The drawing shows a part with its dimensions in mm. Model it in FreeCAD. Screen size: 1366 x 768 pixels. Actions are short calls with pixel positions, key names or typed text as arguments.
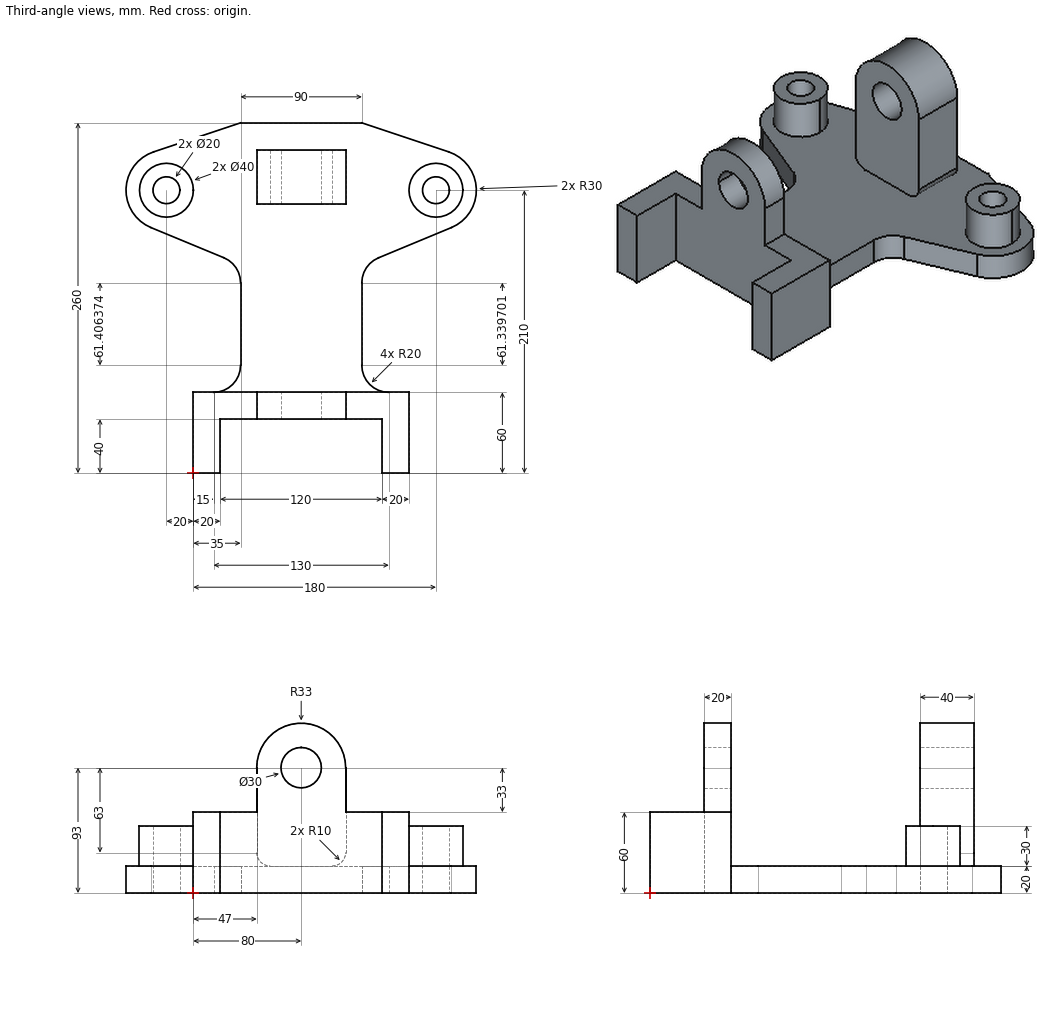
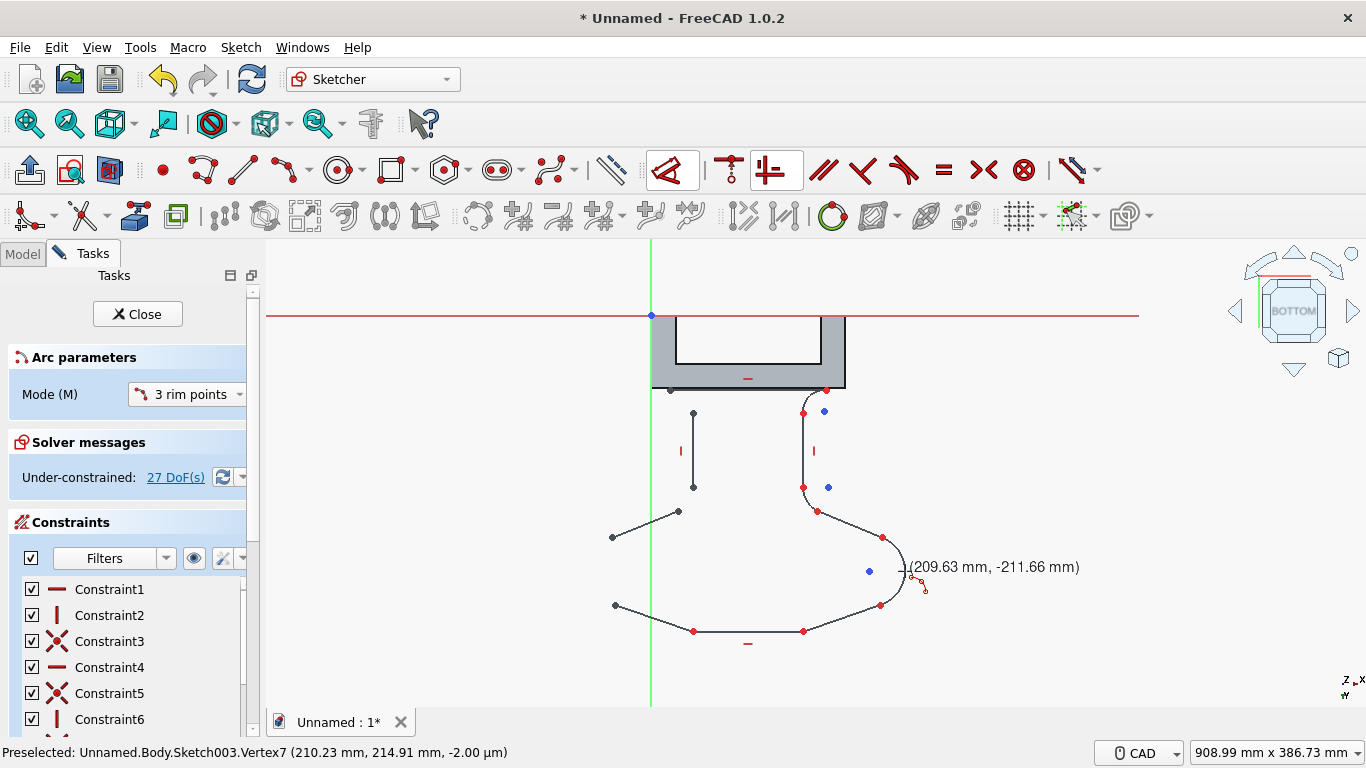
click(615, 605)
click(613, 538)
click(591, 571)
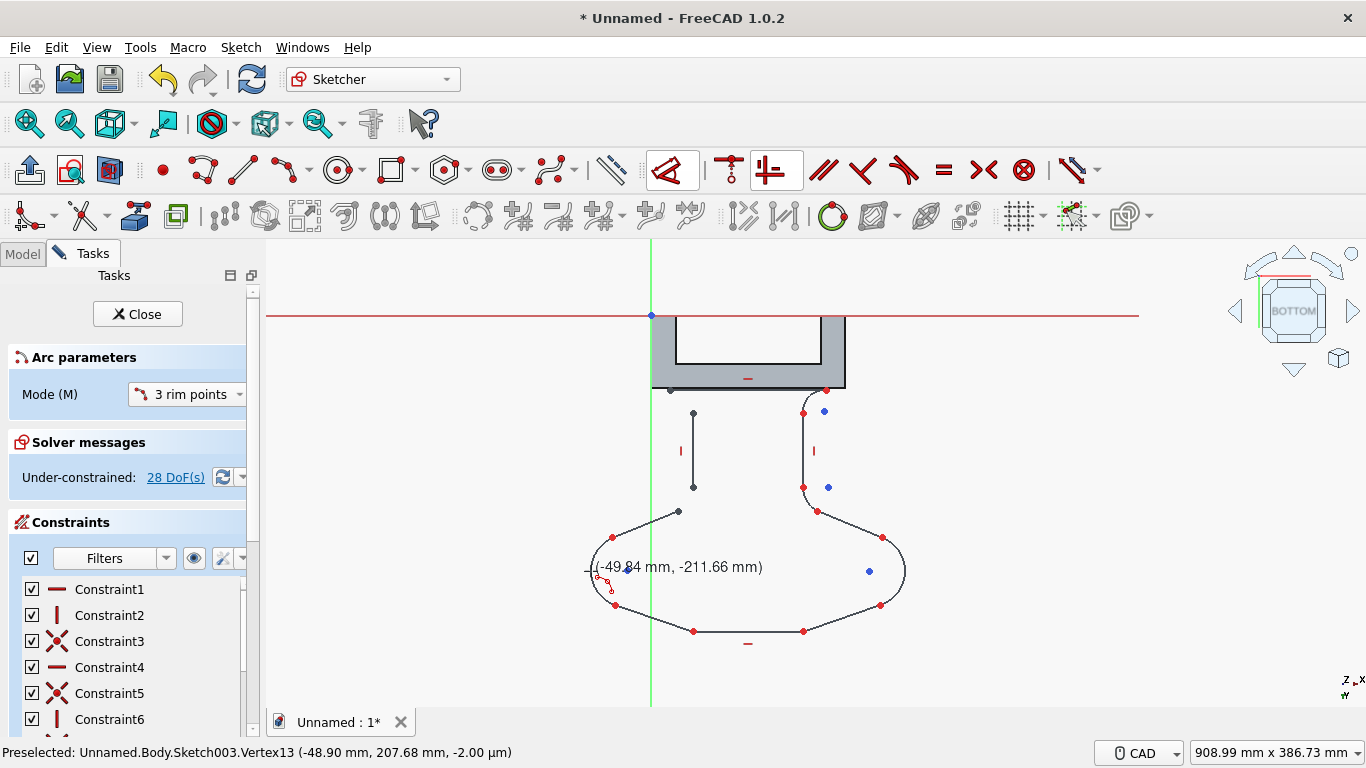
click(679, 511)
click(693, 488)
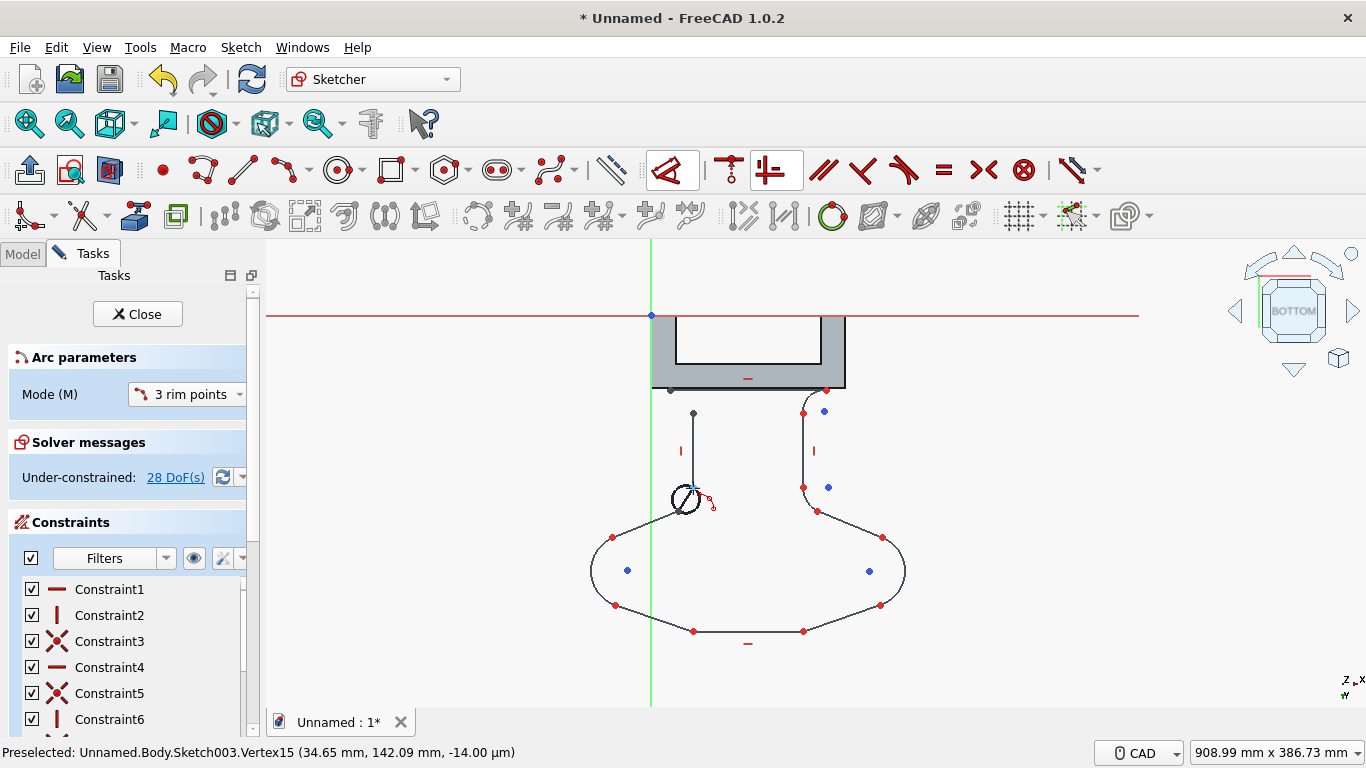
scroll(690, 500, up, 7)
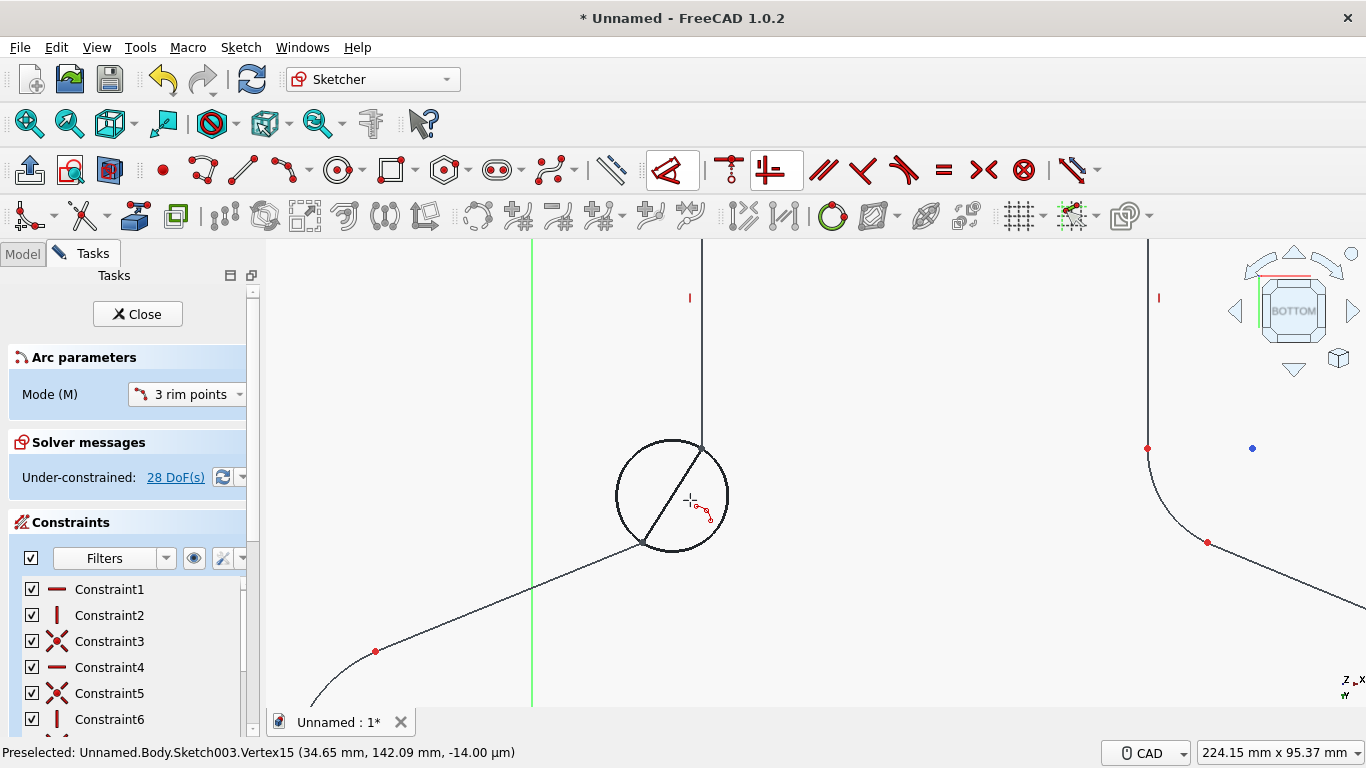
click(687, 500)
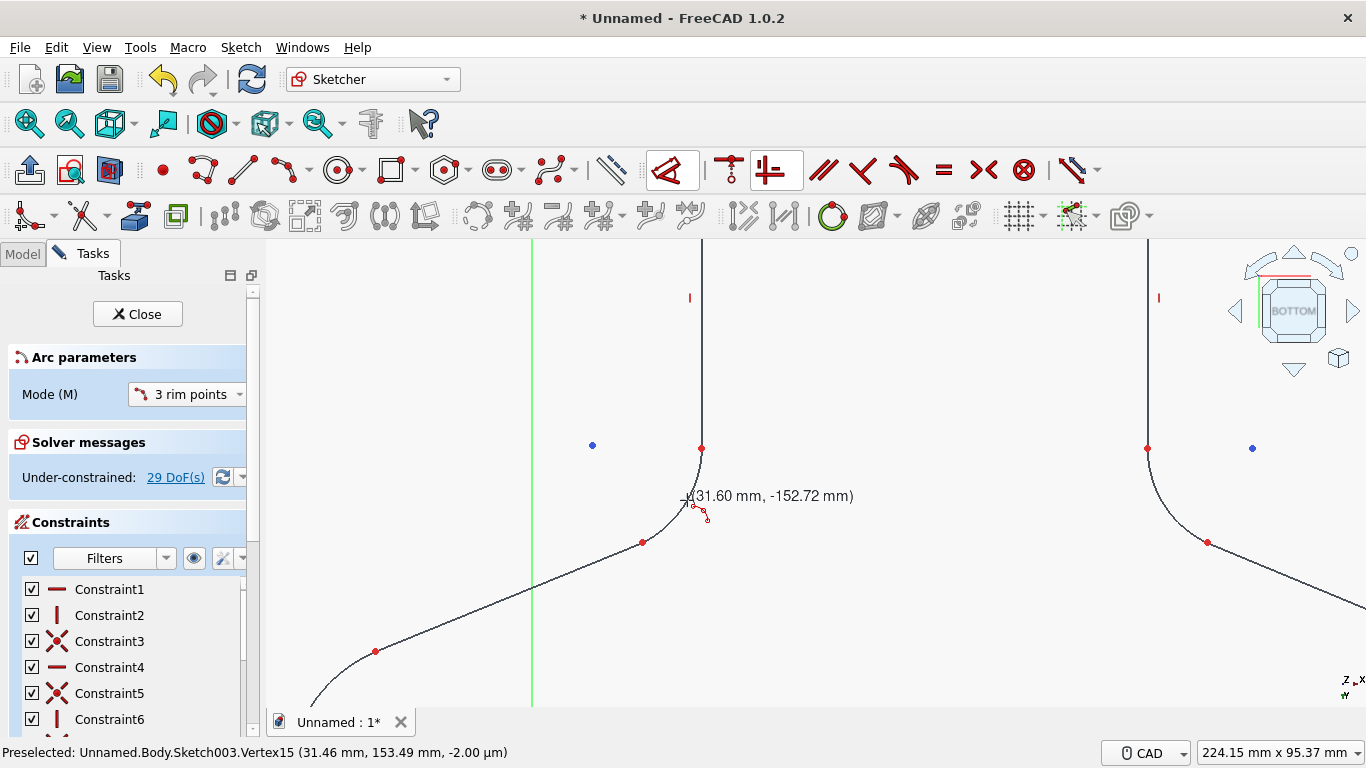
scroll(690, 500, down, 7)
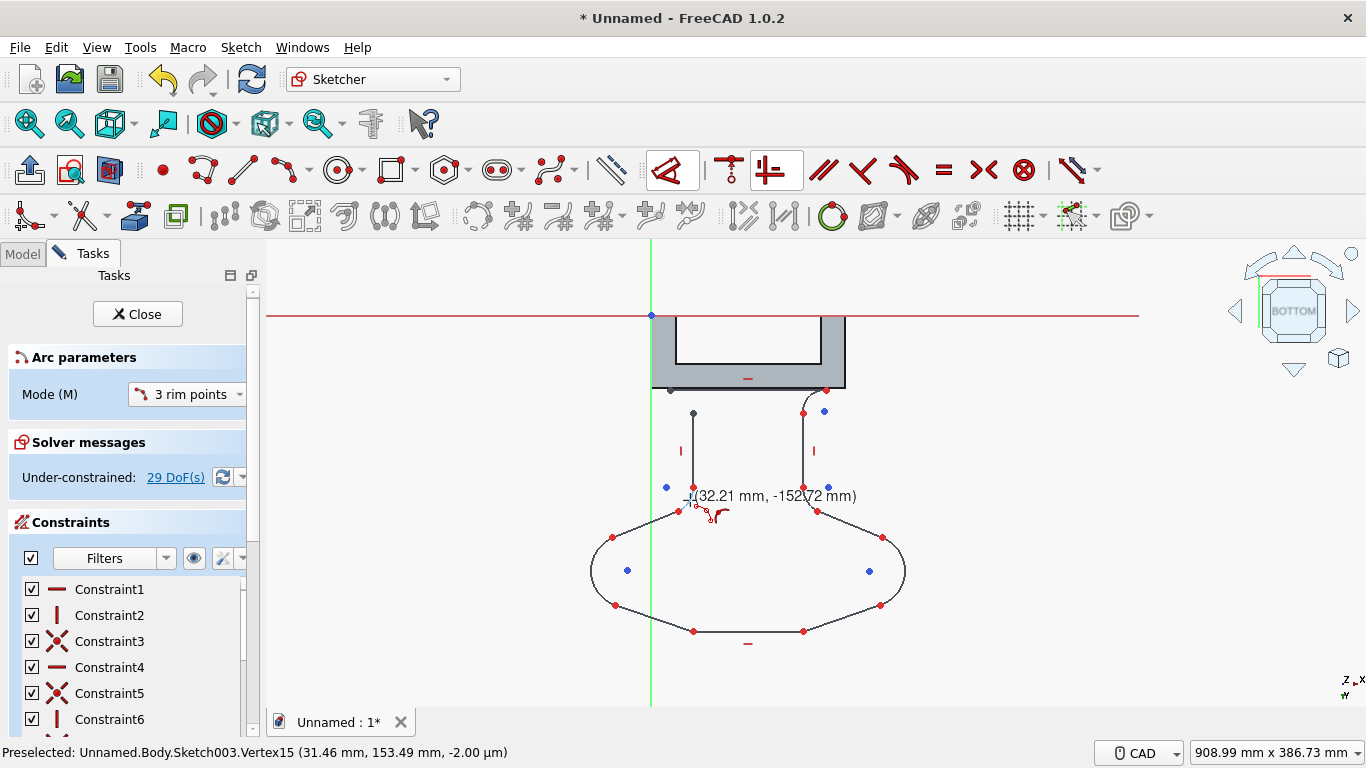
click(693, 413)
click(670, 390)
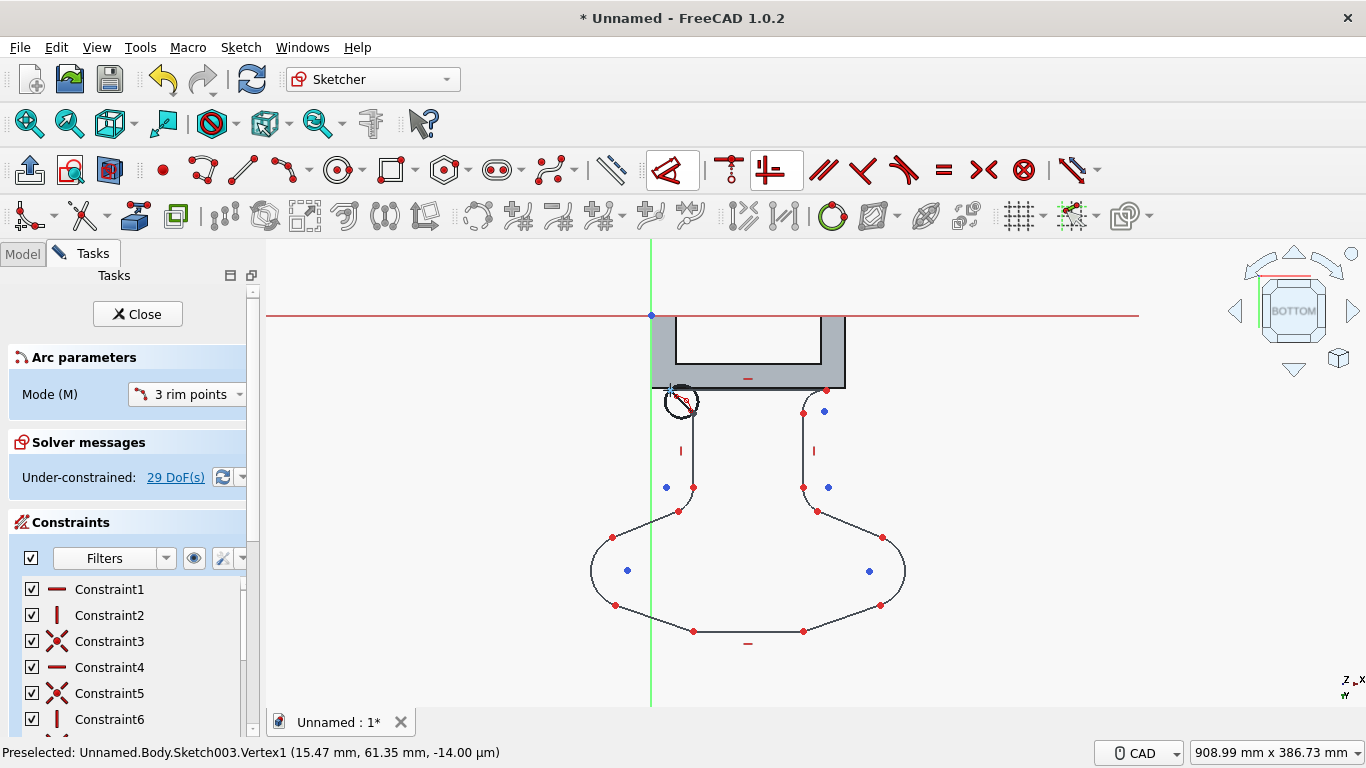
scroll(687, 396, up, 5)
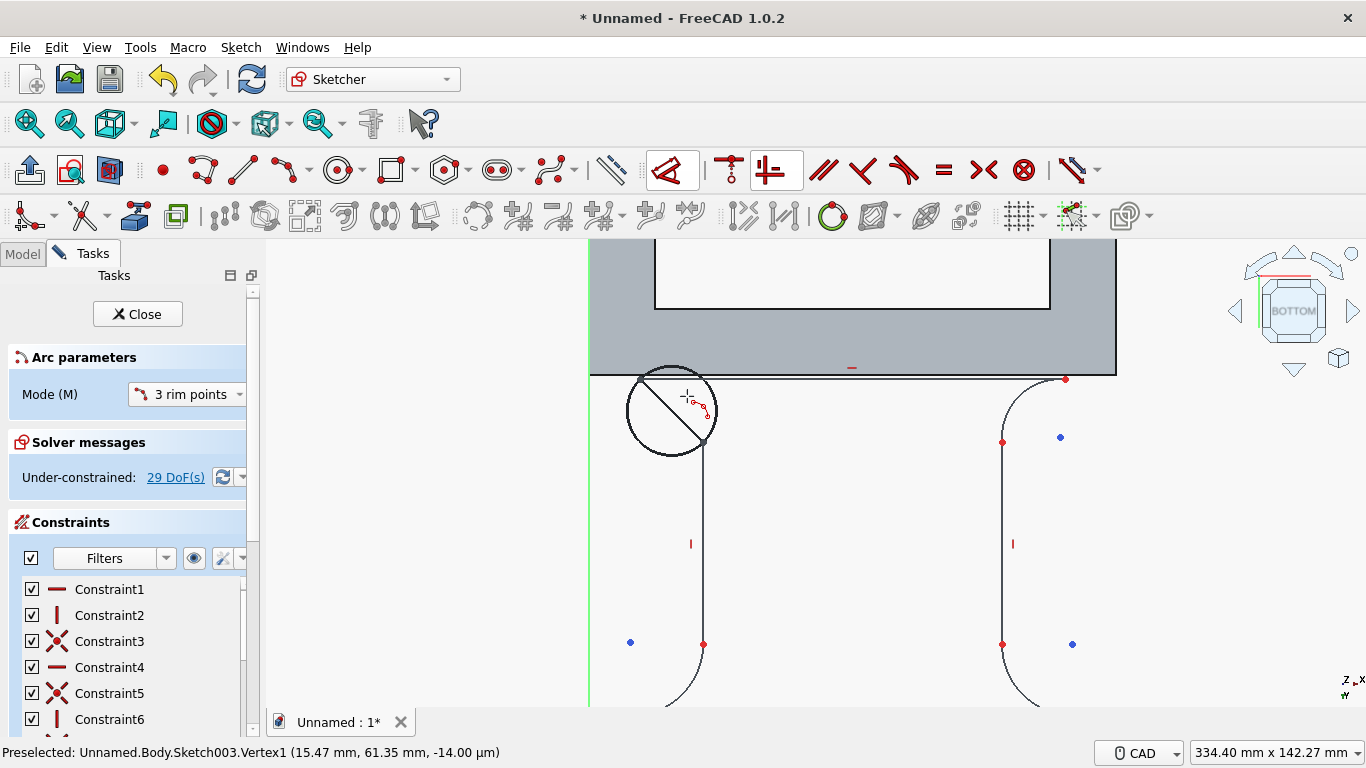
click(685, 394)
key(Escape)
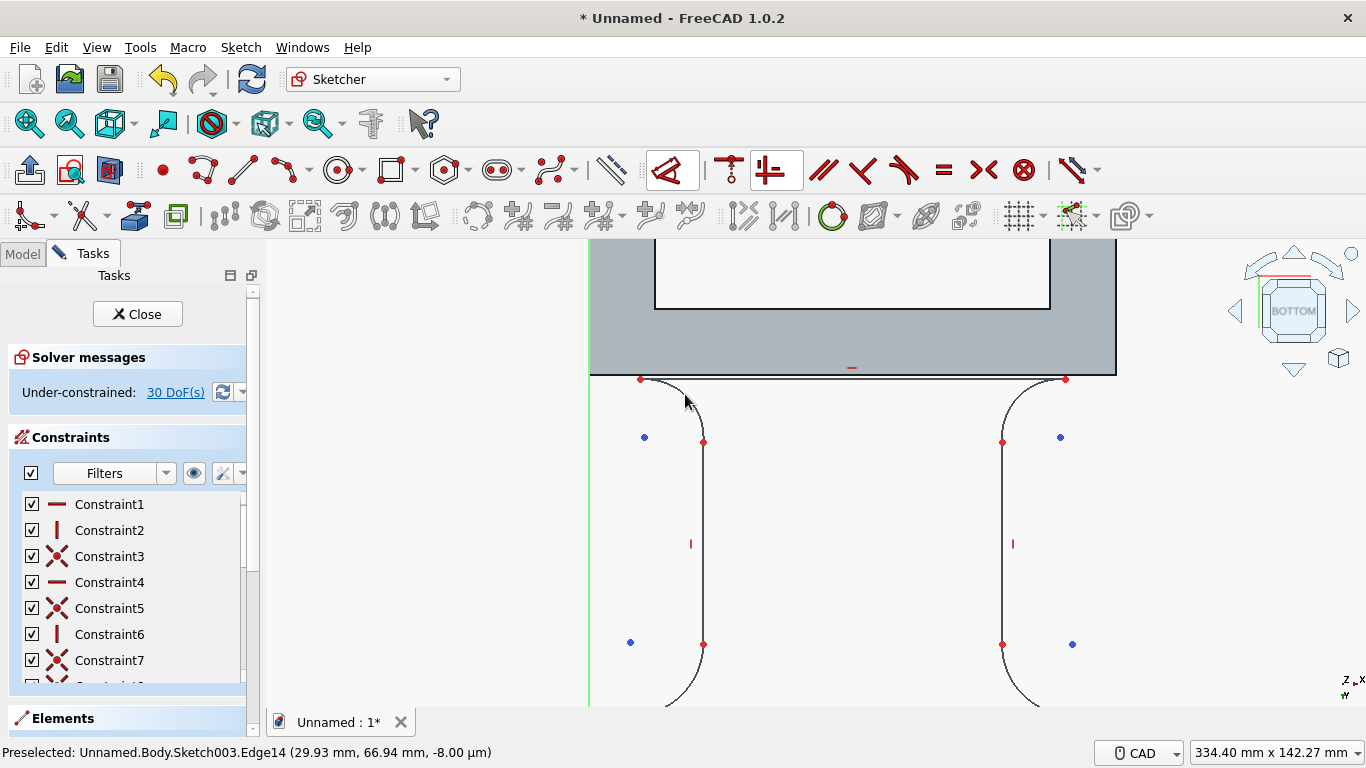
click(768, 379)